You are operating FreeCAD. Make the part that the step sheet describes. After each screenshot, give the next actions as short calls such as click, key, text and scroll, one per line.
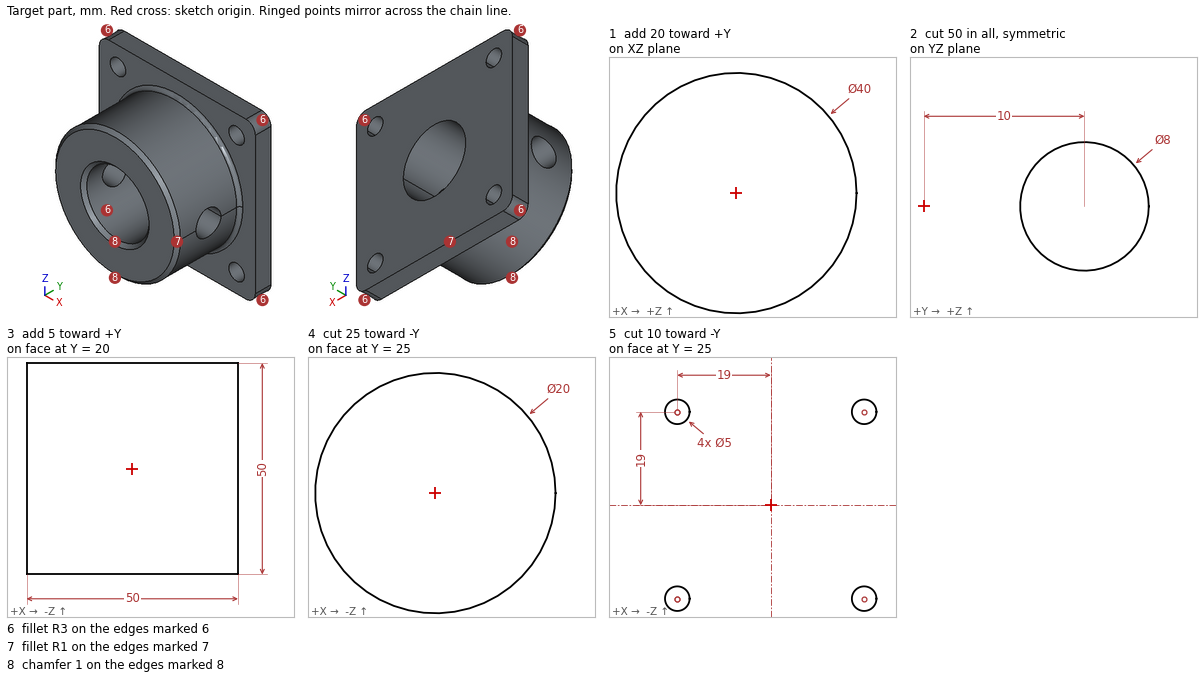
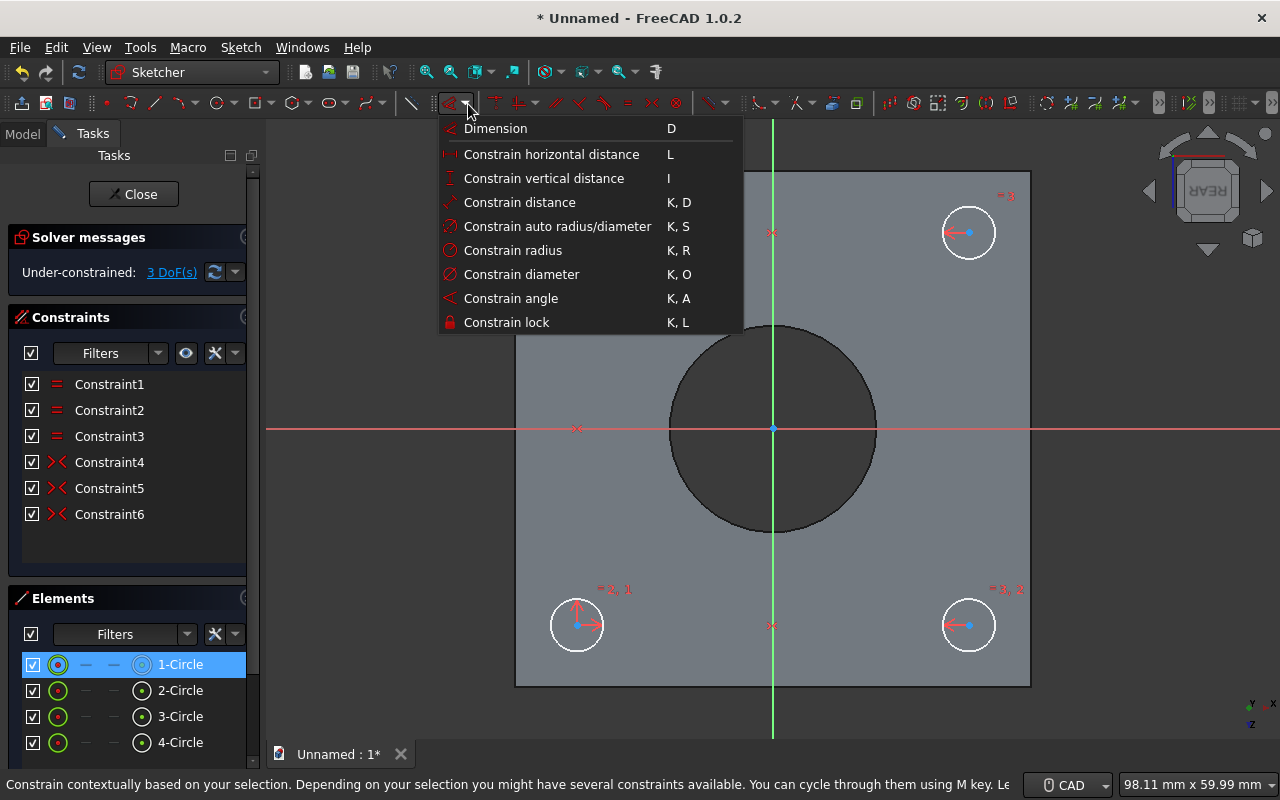
click(591, 274)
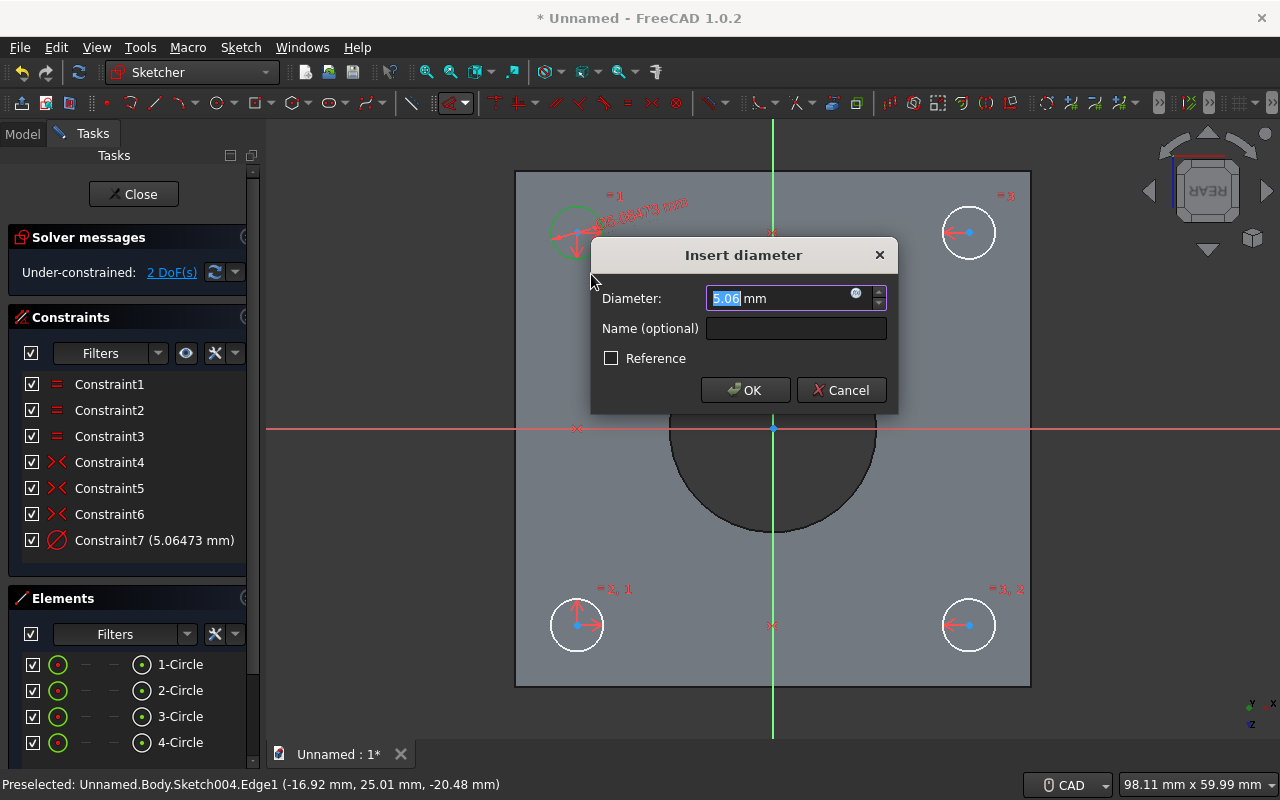
text(5)
key(Return)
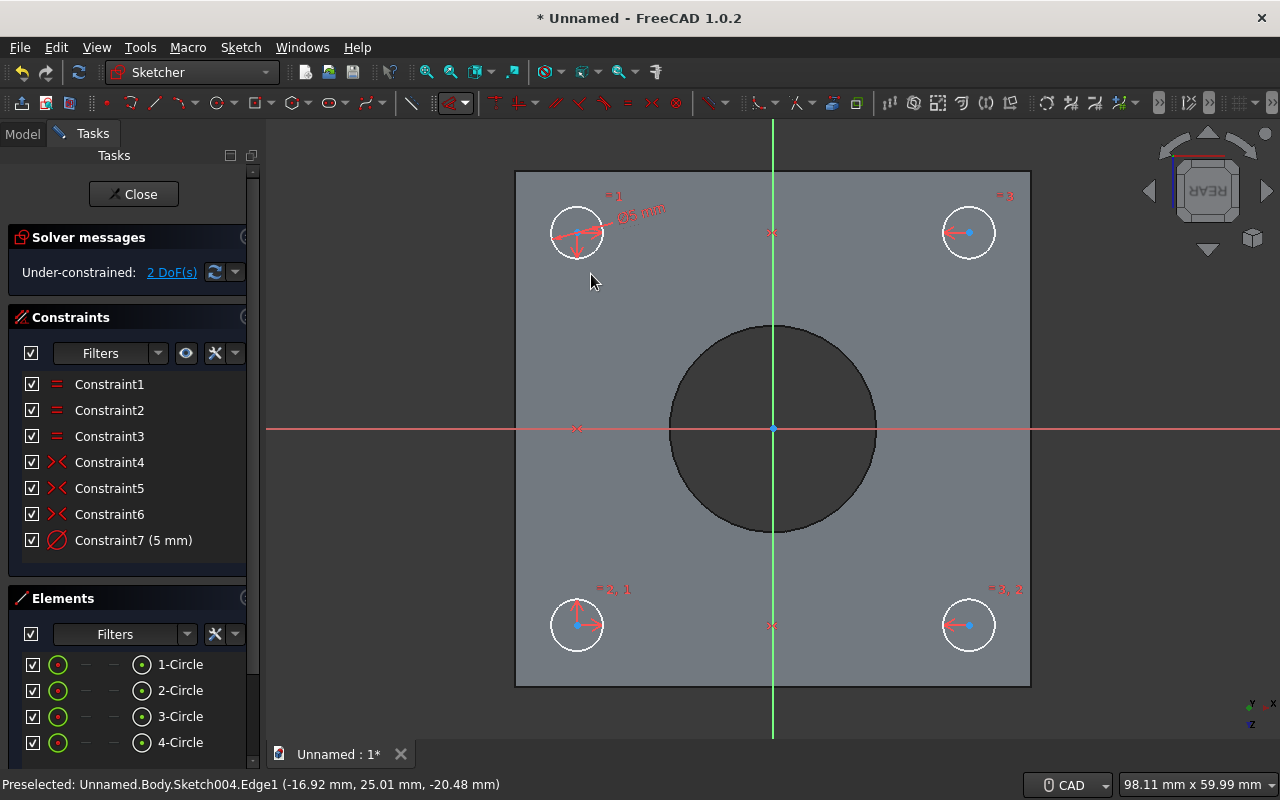
click(577, 233)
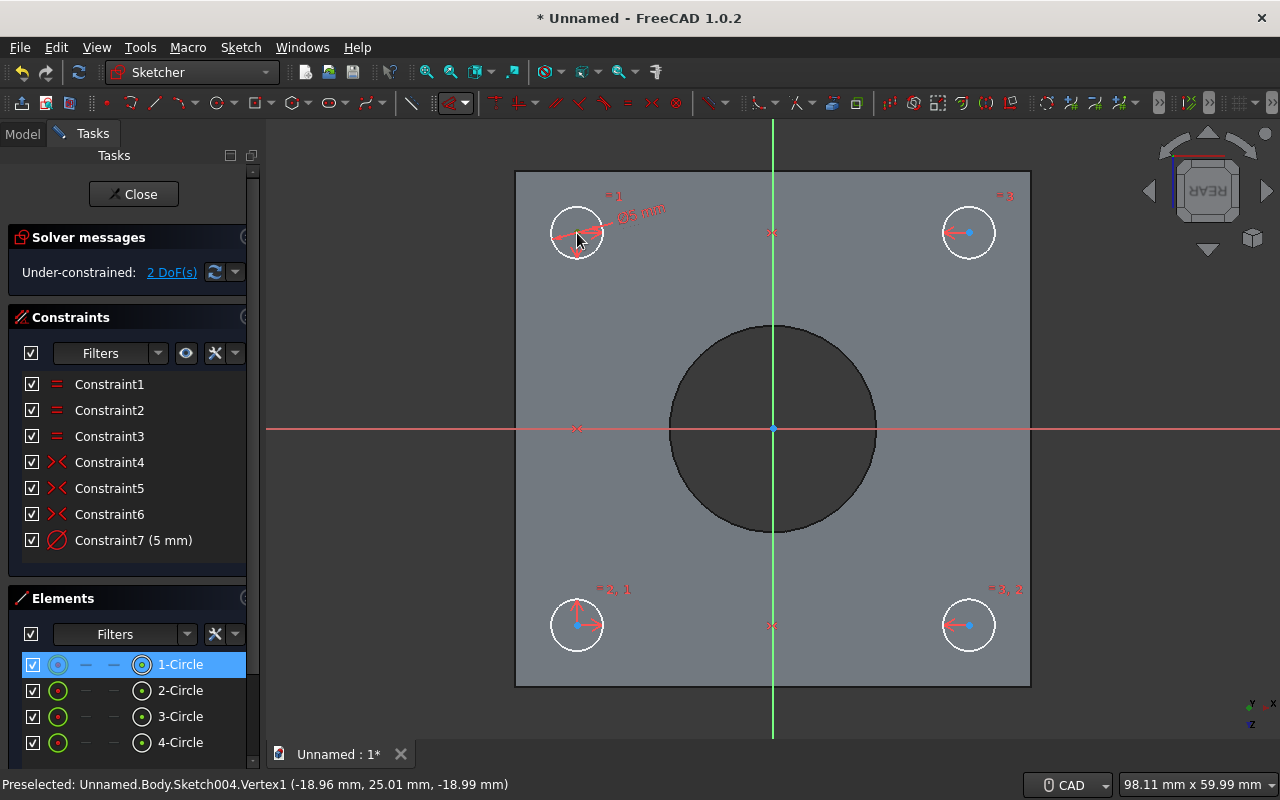
click(468, 104)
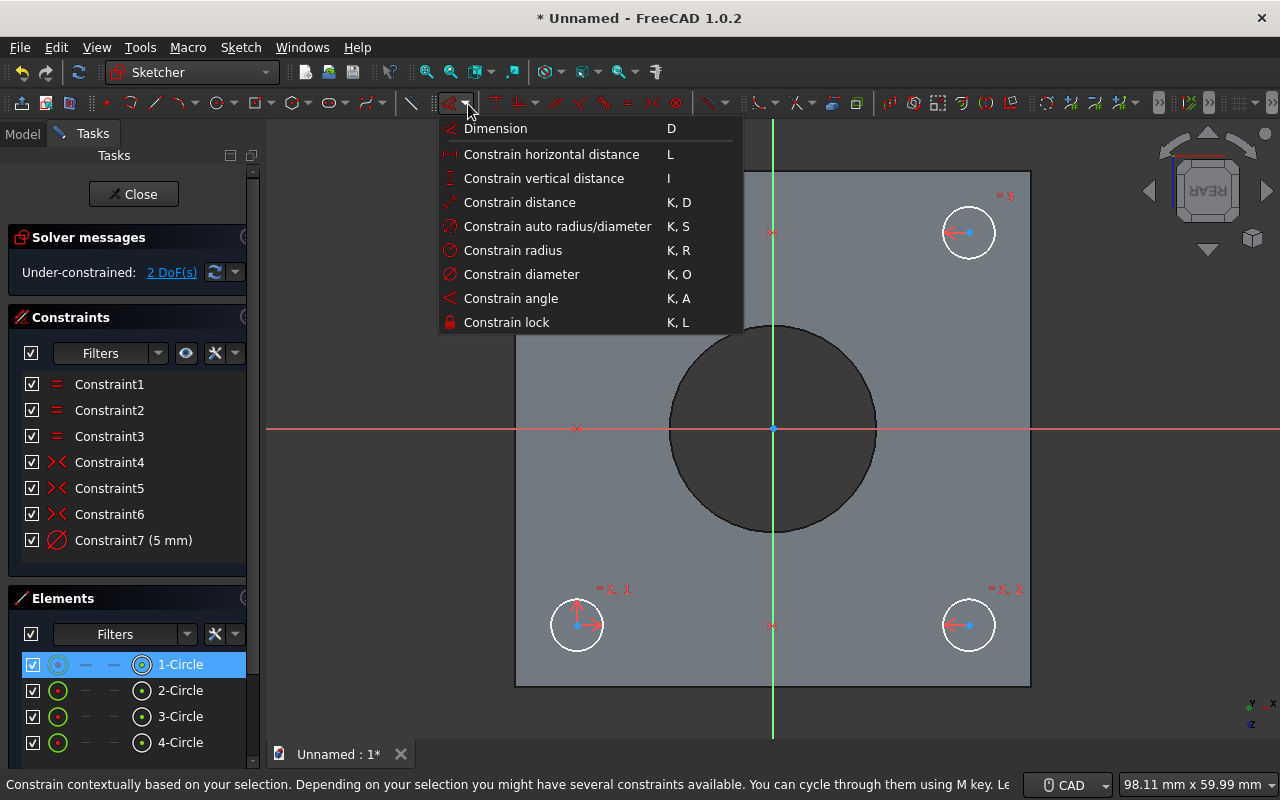
click(591, 154)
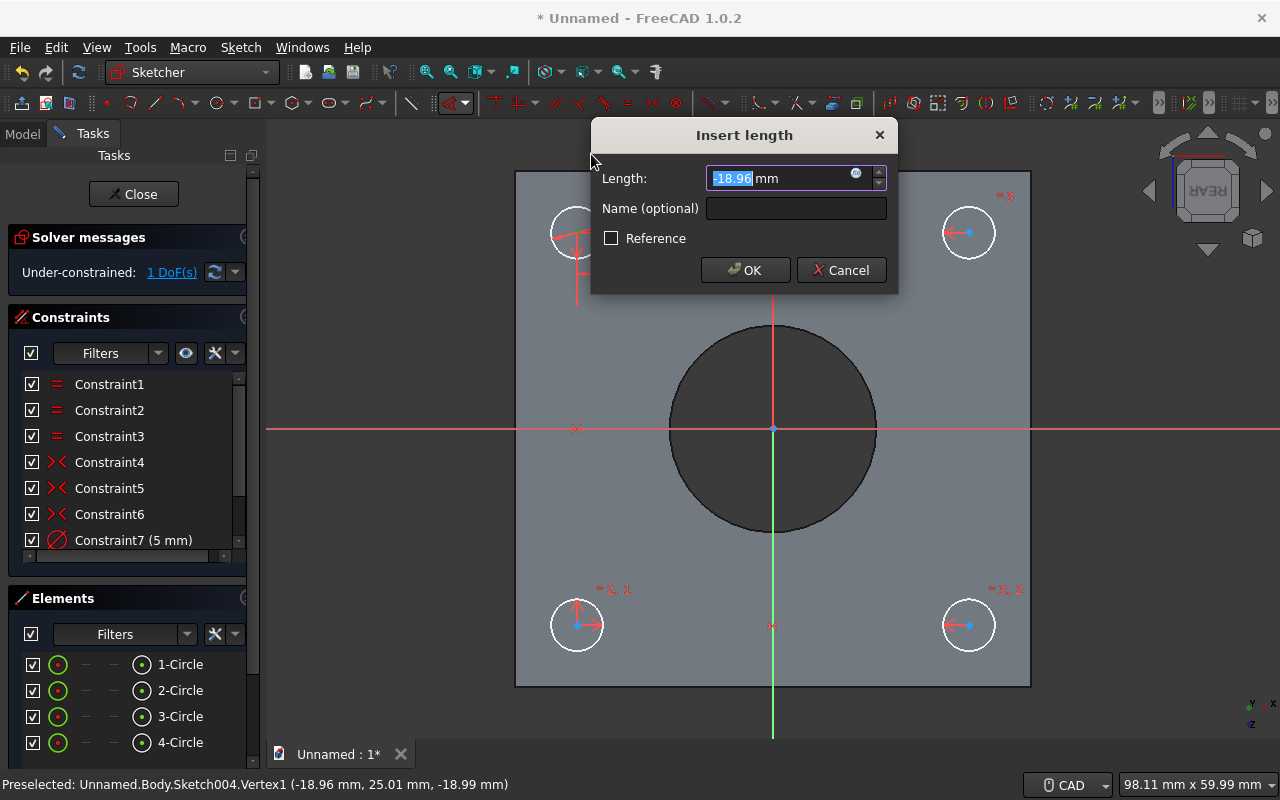
text(-19)
key(Return)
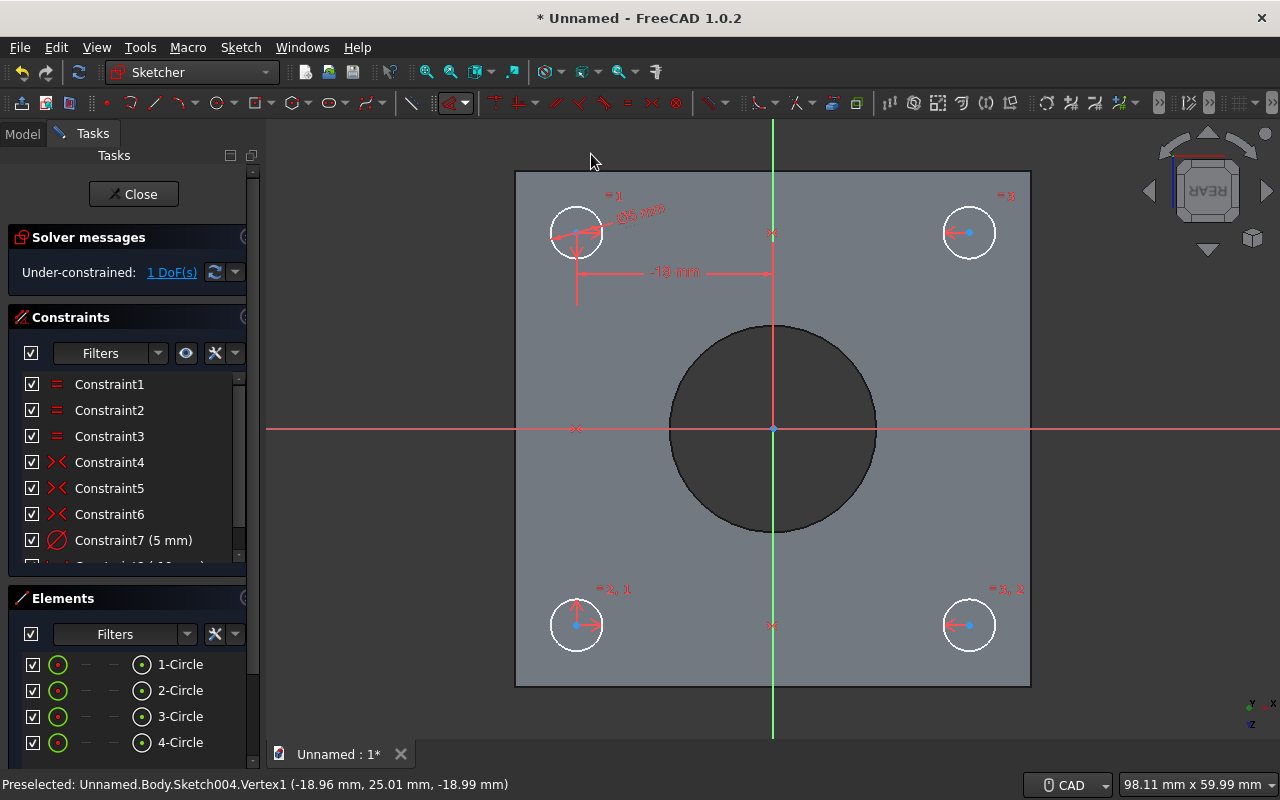
click(577, 233)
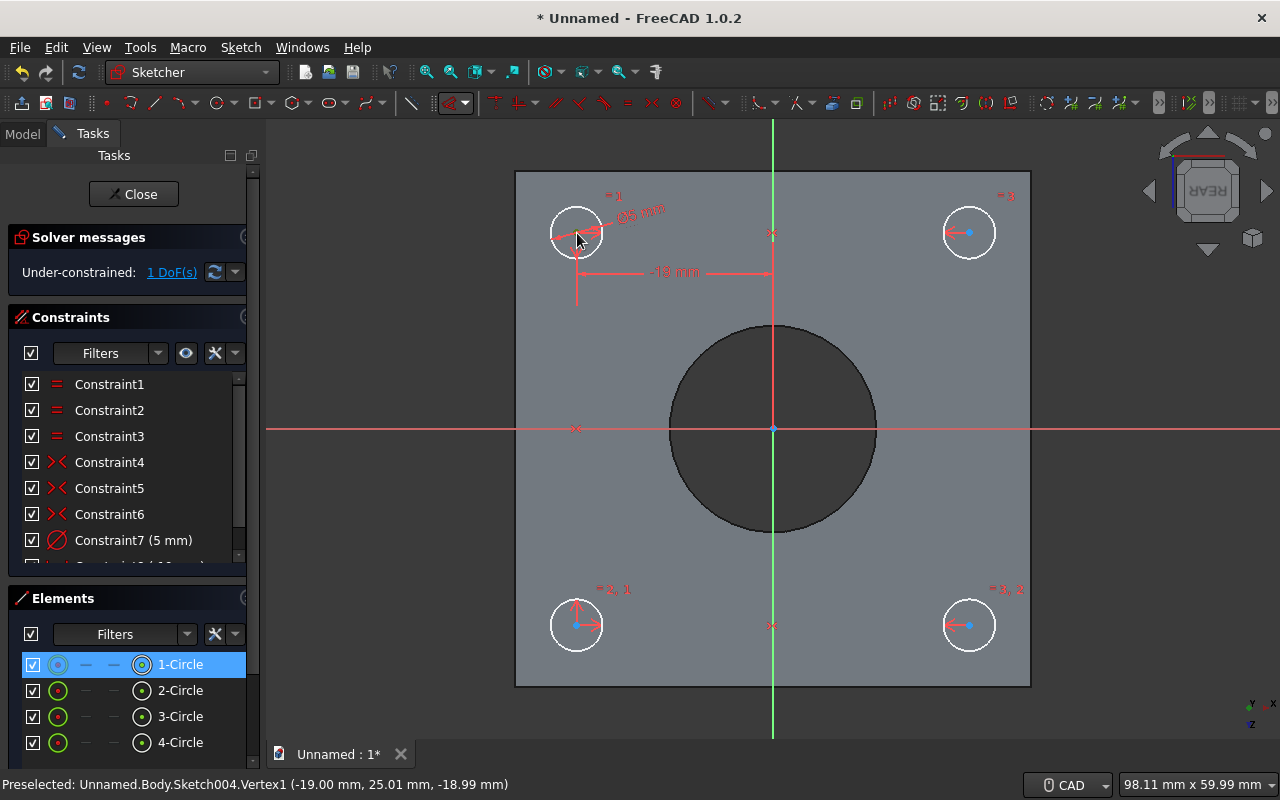
click(468, 104)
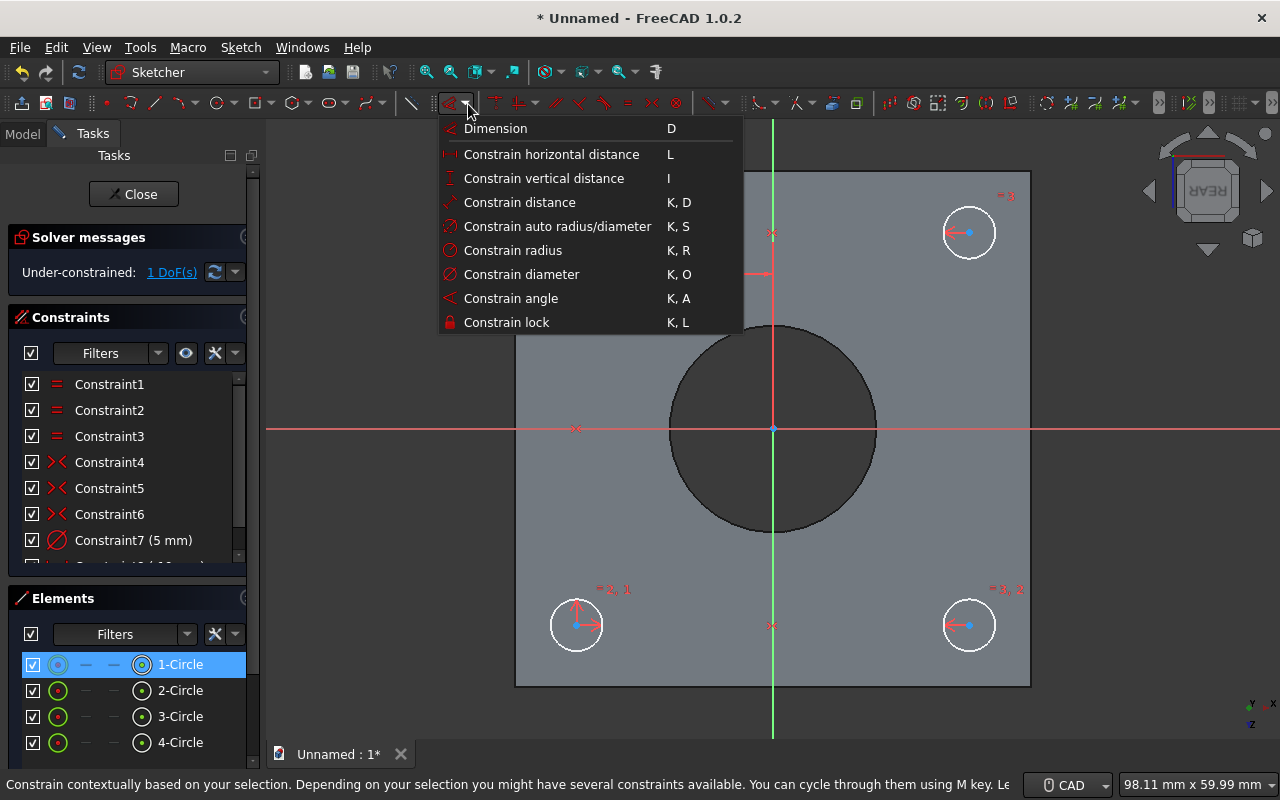
click(591, 178)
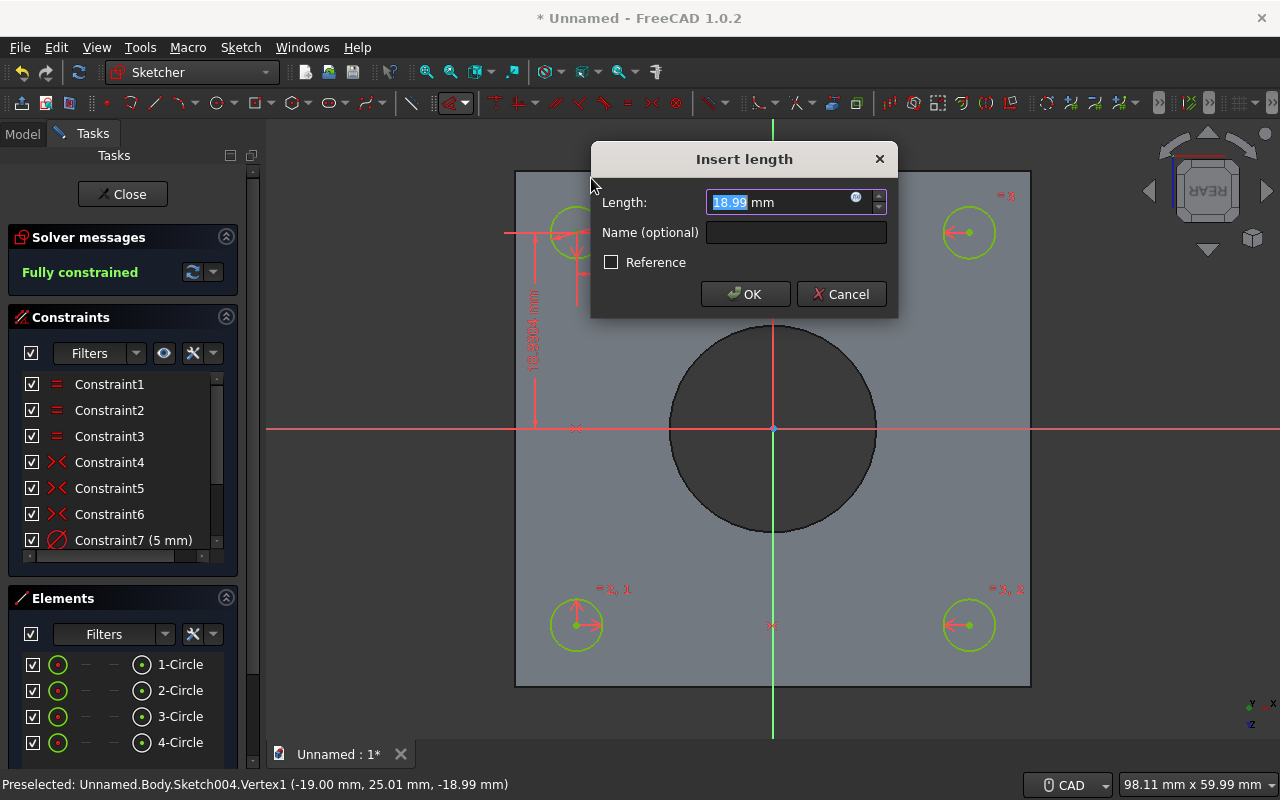
text(19)
key(Return)